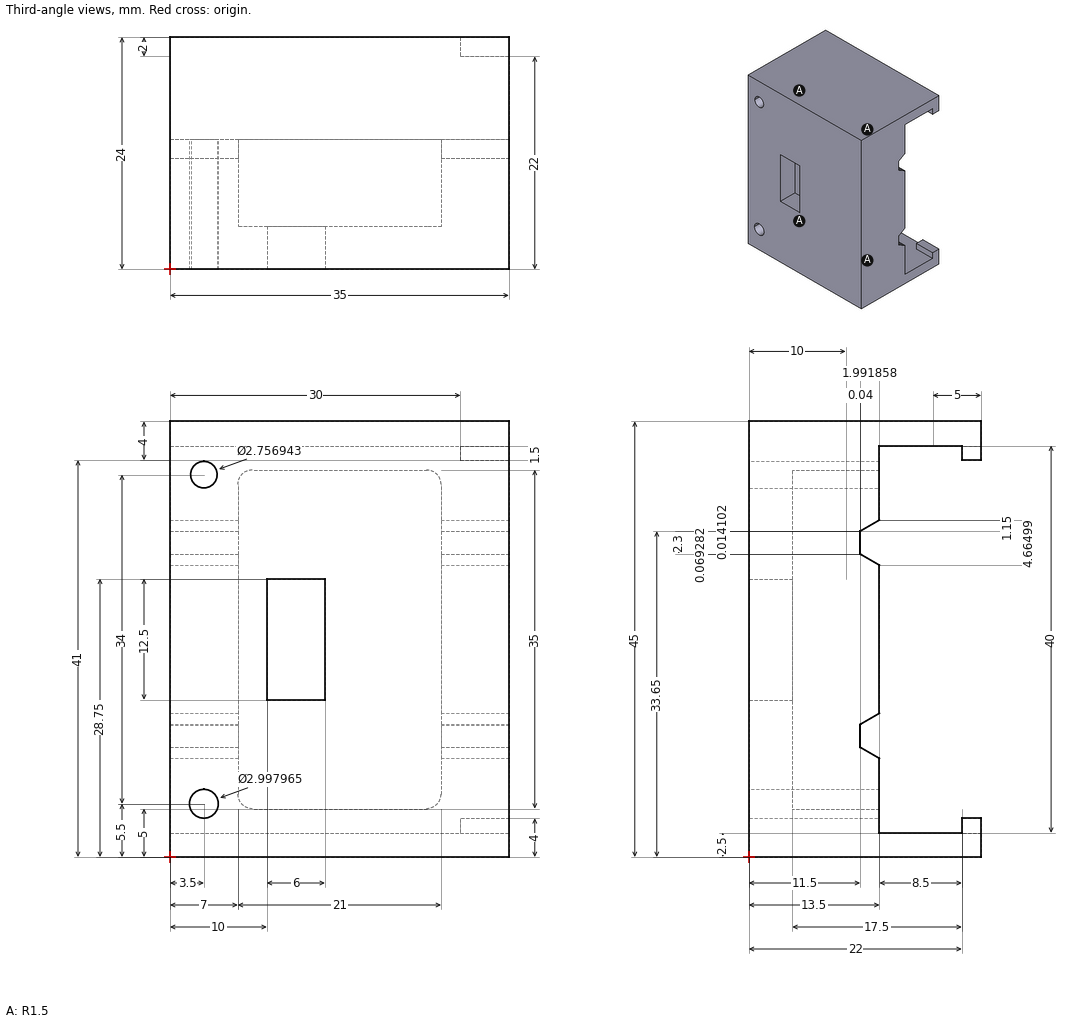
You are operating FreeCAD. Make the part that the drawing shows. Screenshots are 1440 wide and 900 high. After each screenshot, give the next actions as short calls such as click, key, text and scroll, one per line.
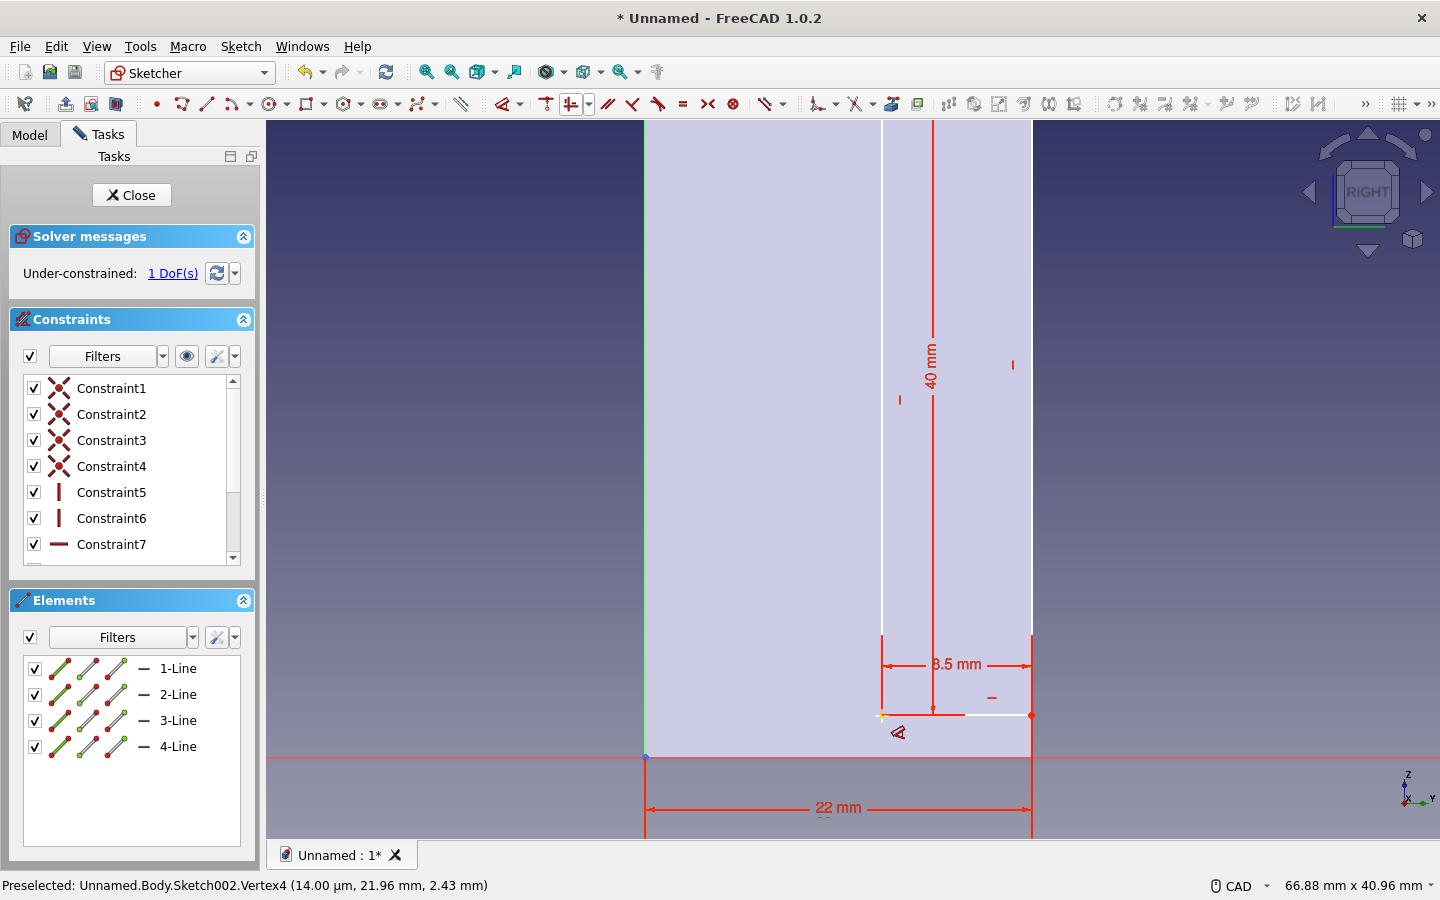
click(882, 715)
click(611, 736)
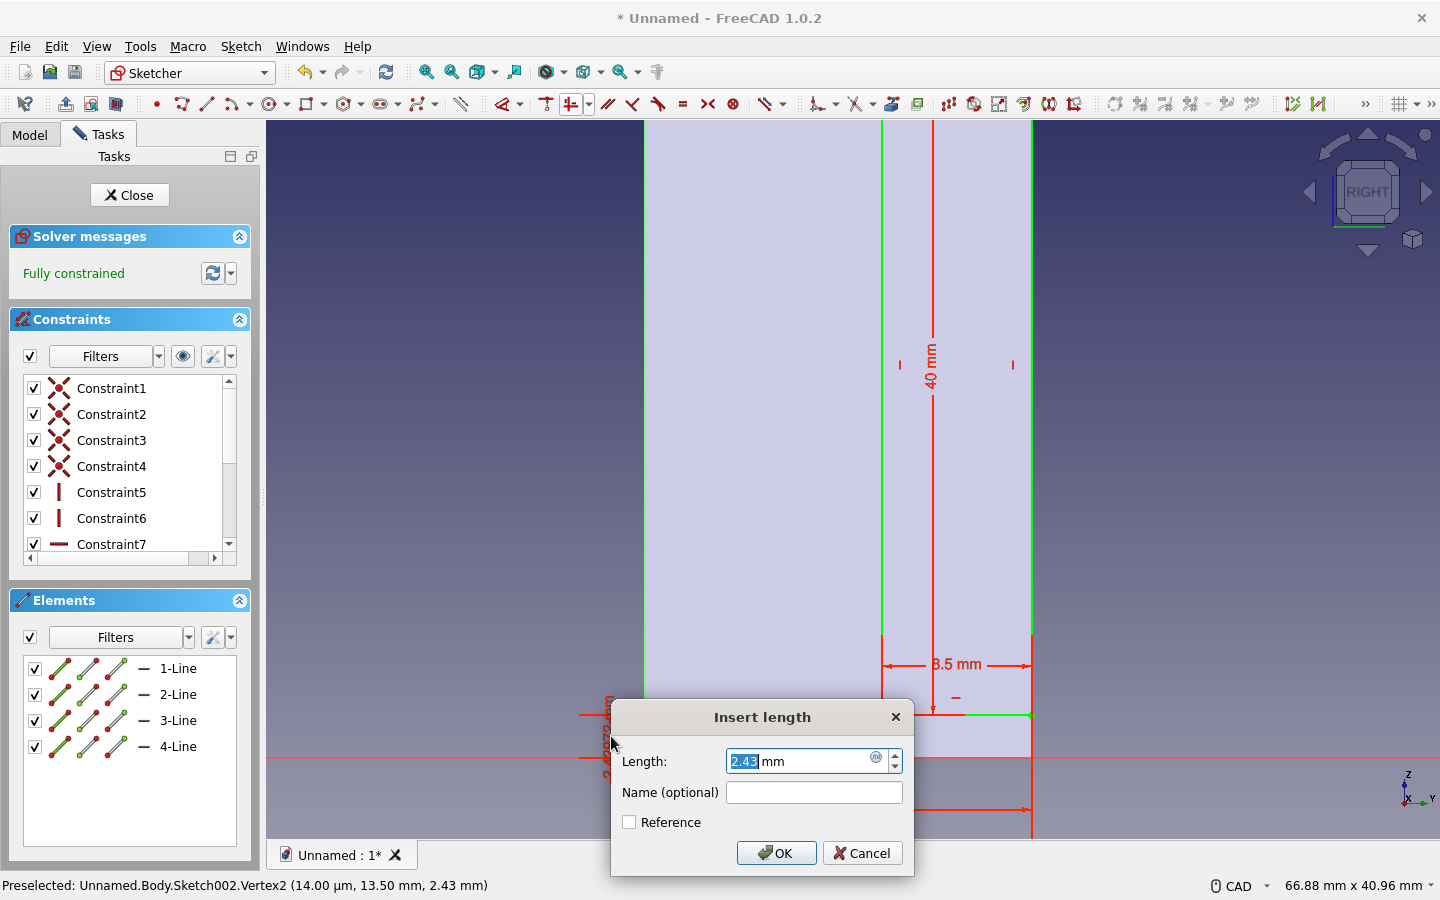
text(2.5)
key(Return)
key(Escape)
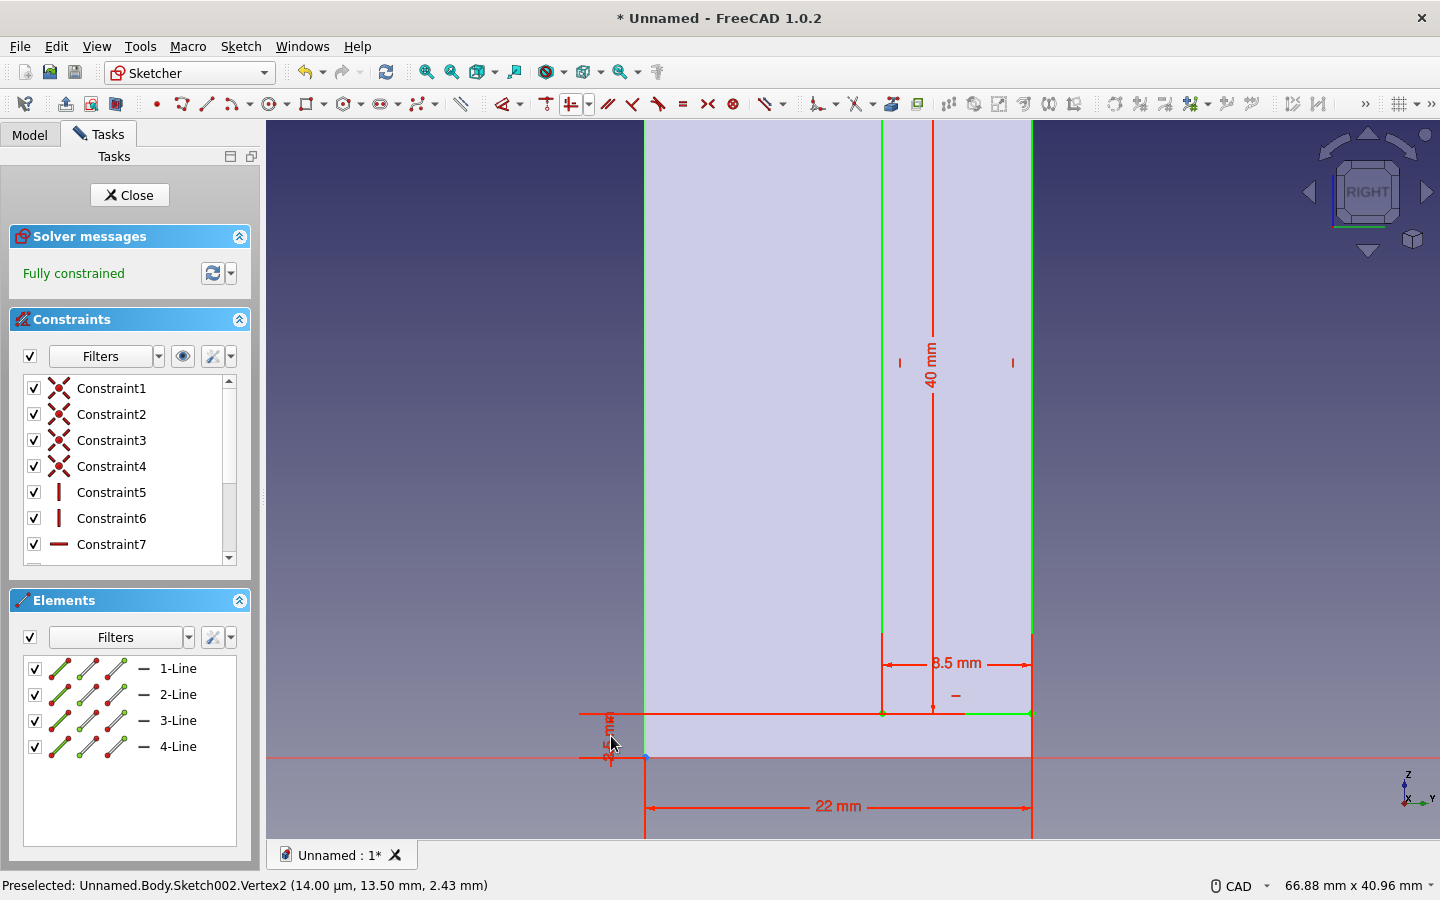
click(130, 195)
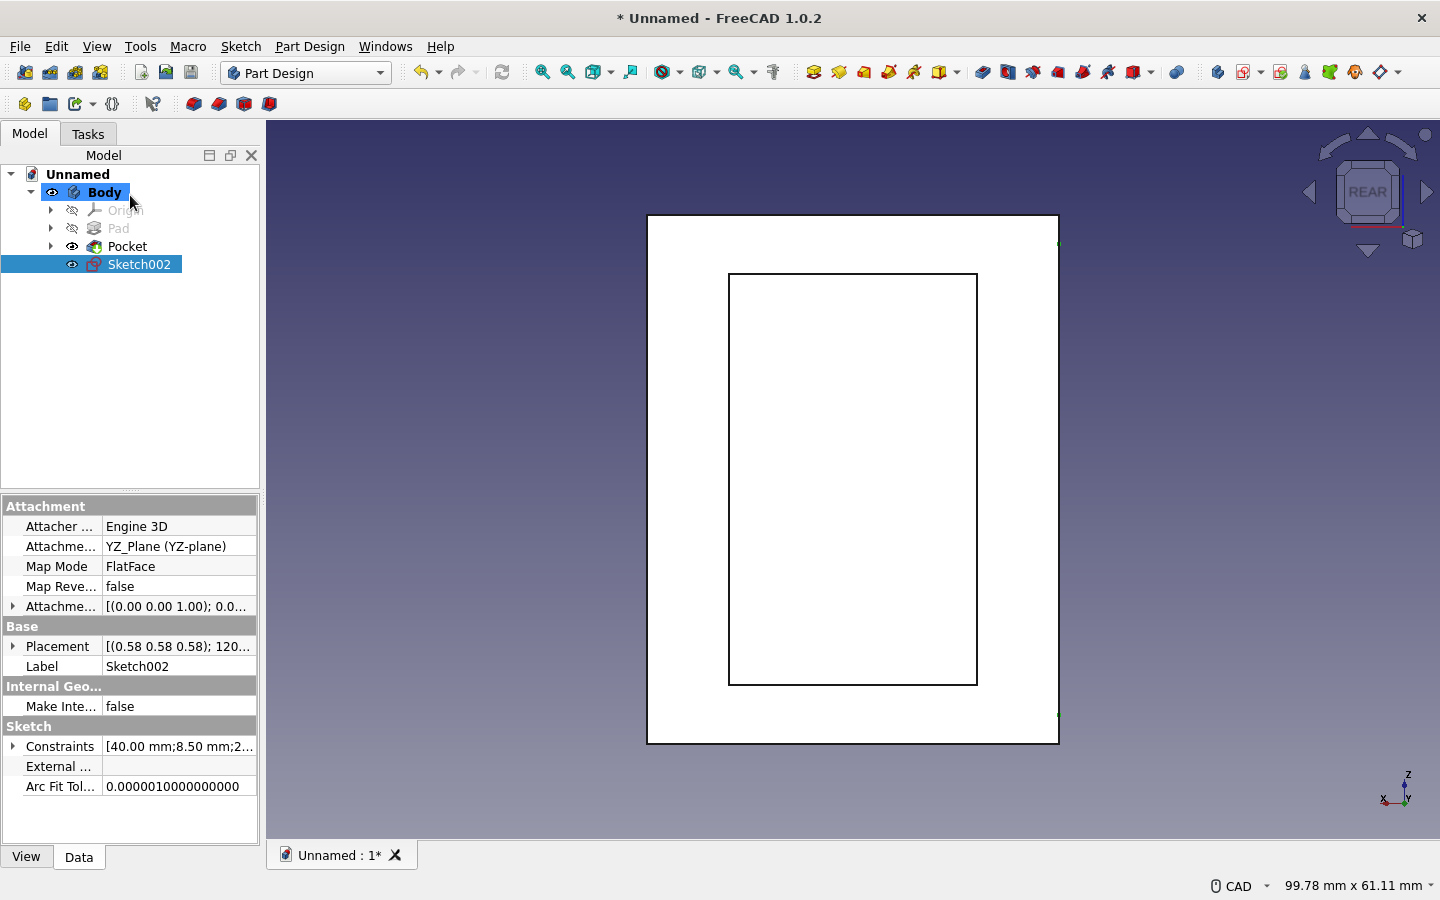
click(983, 72)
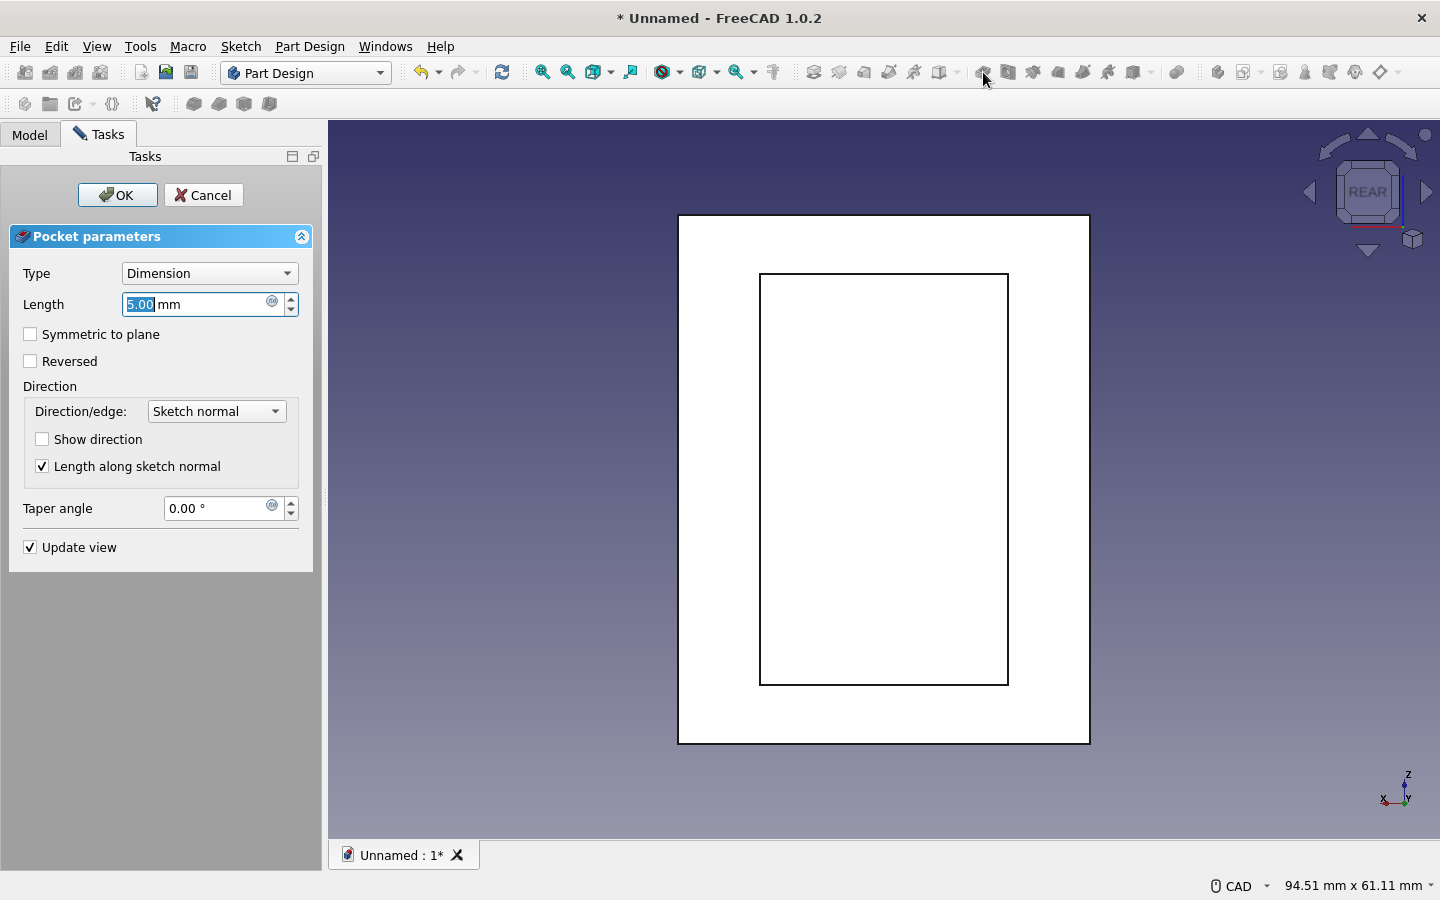
click(210, 274)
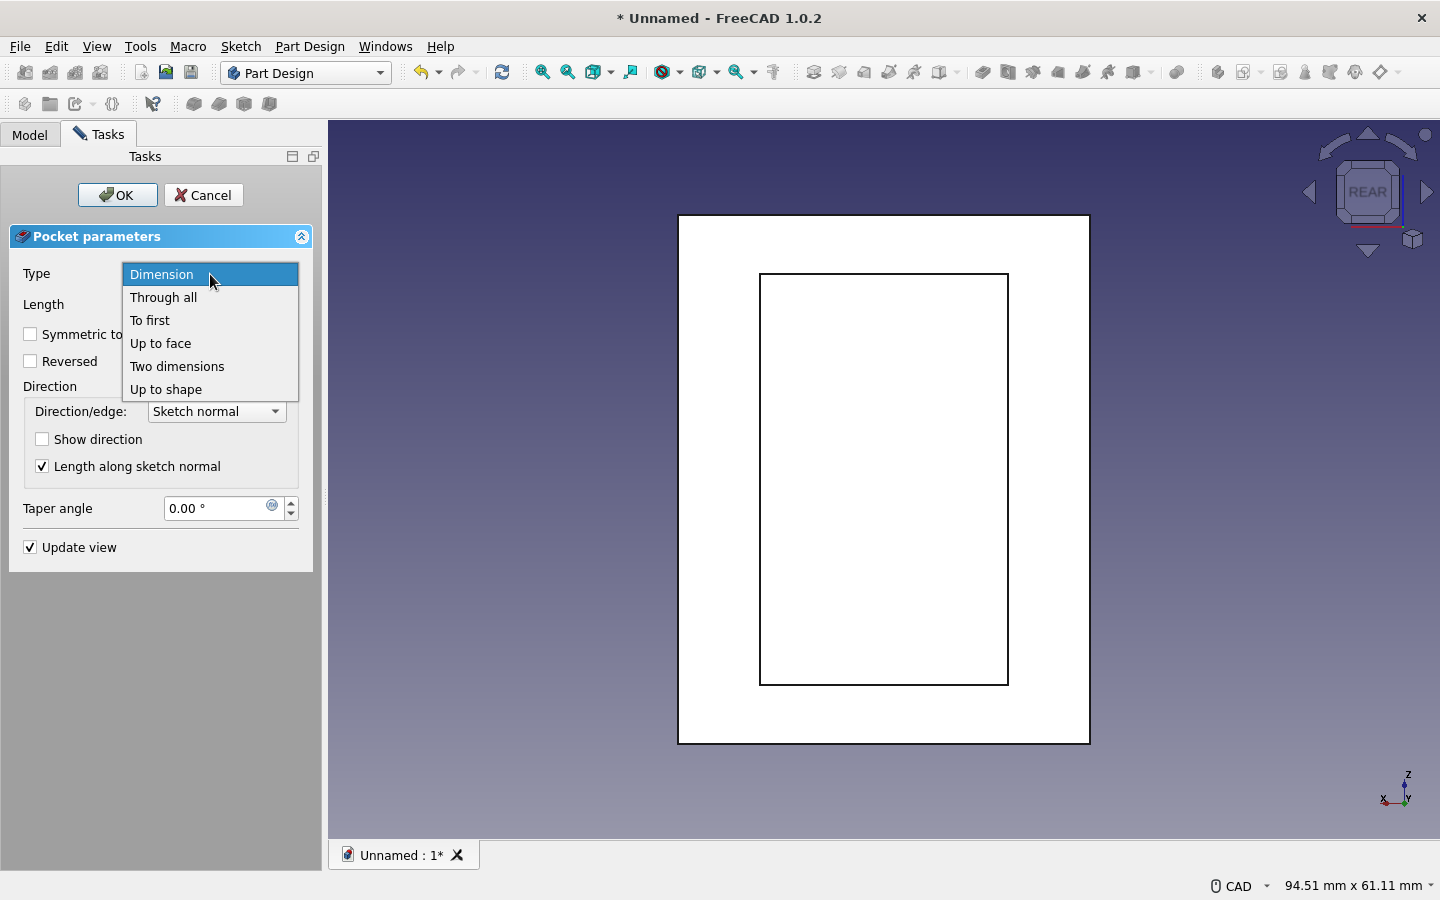
click(208, 298)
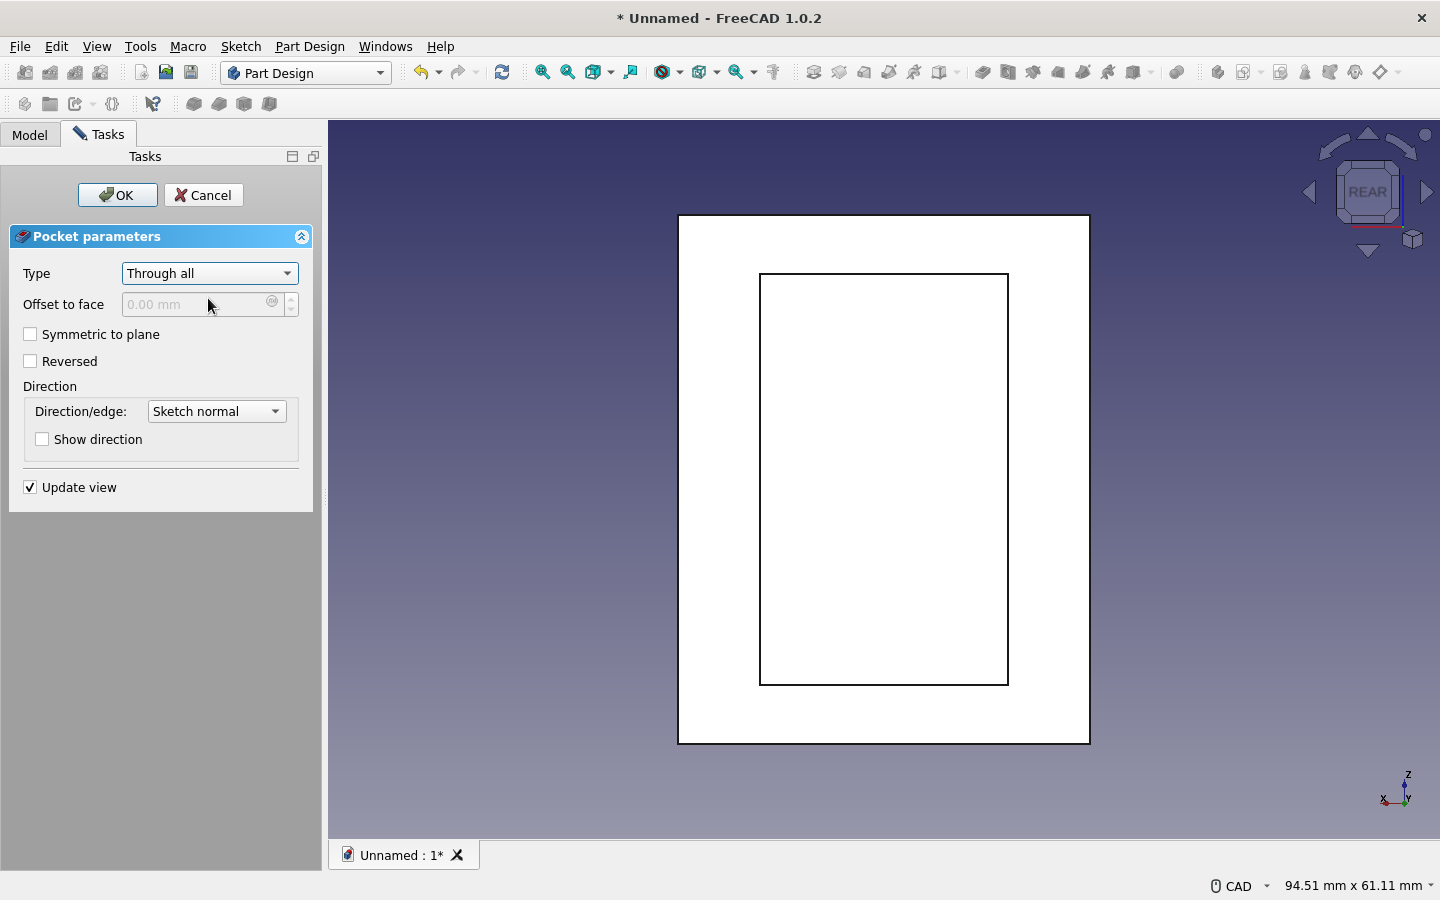
click(31, 361)